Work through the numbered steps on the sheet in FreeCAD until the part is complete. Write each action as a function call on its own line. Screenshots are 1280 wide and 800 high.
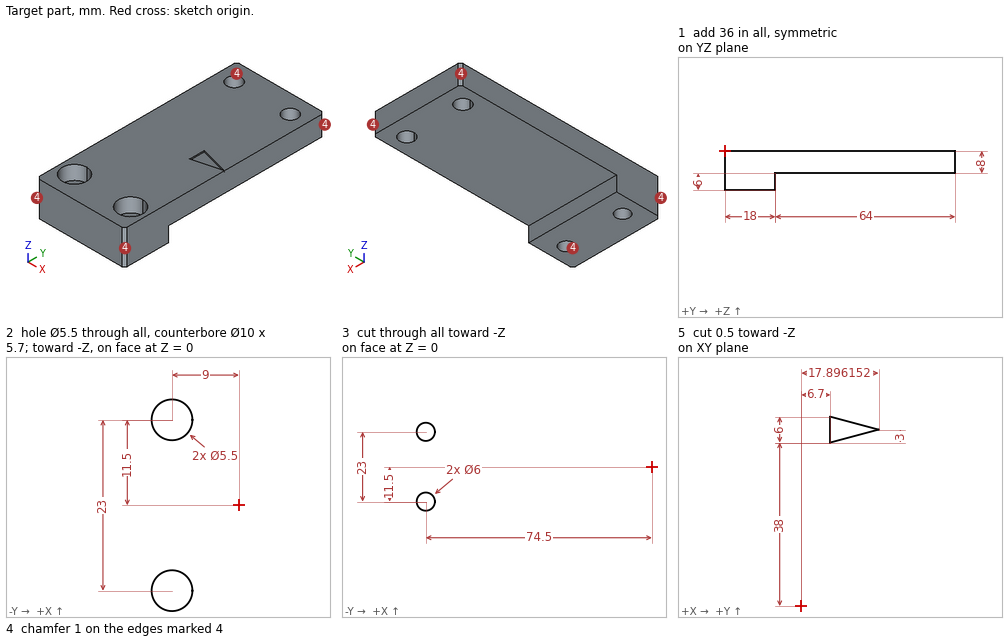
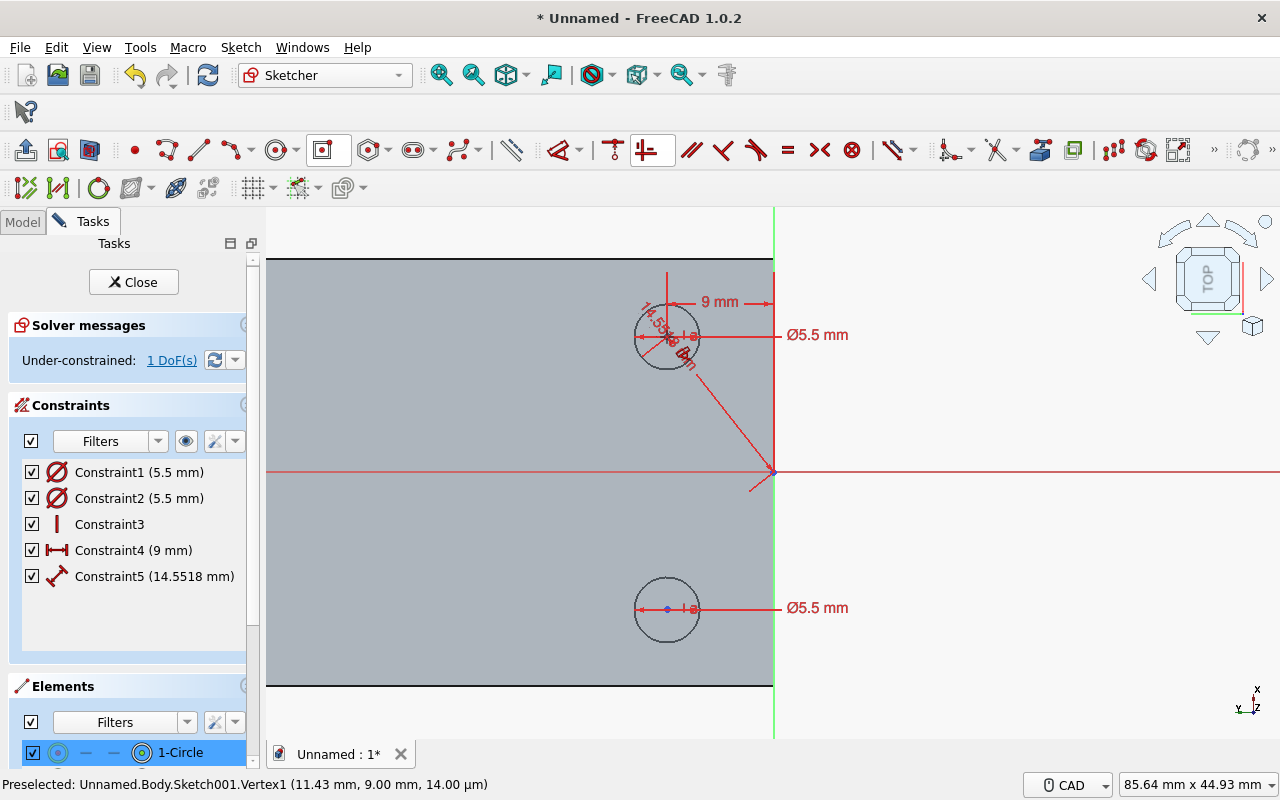
click(667, 610)
click(633, 411)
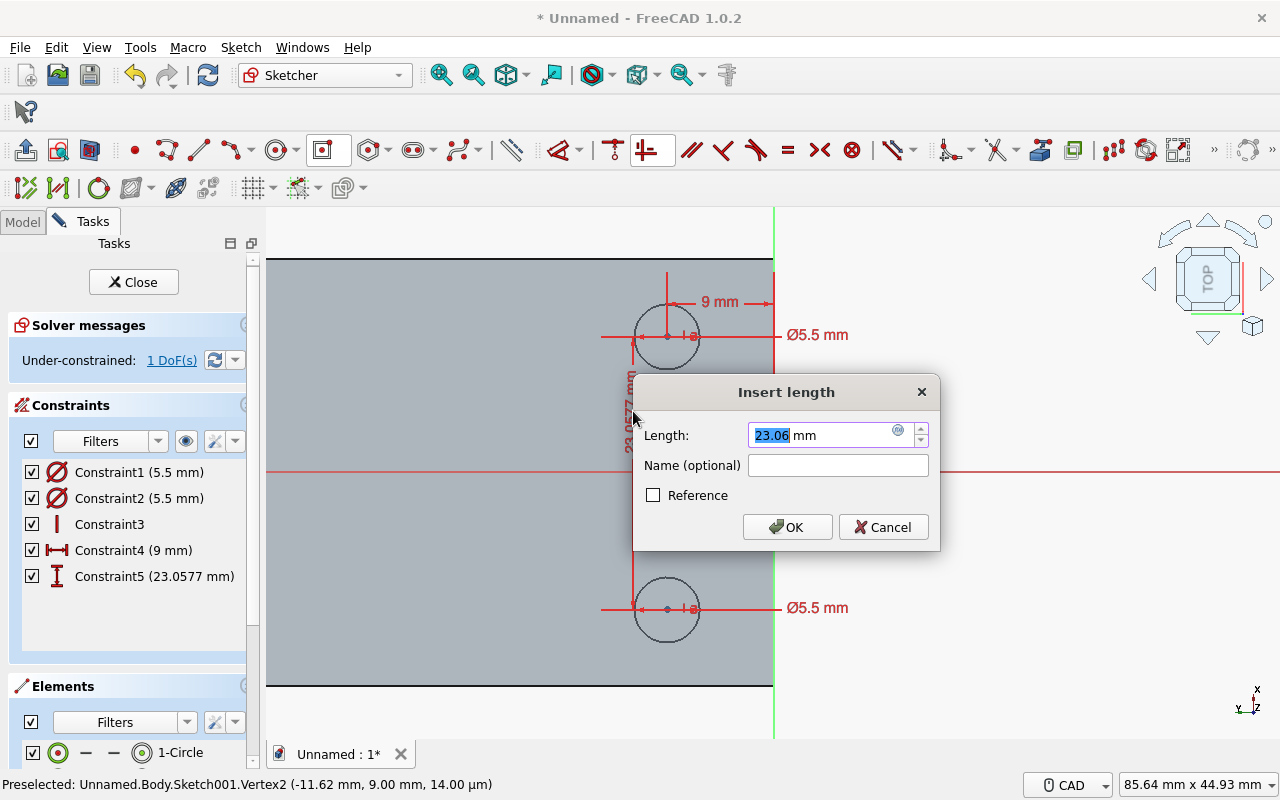
text(23)
key(Return)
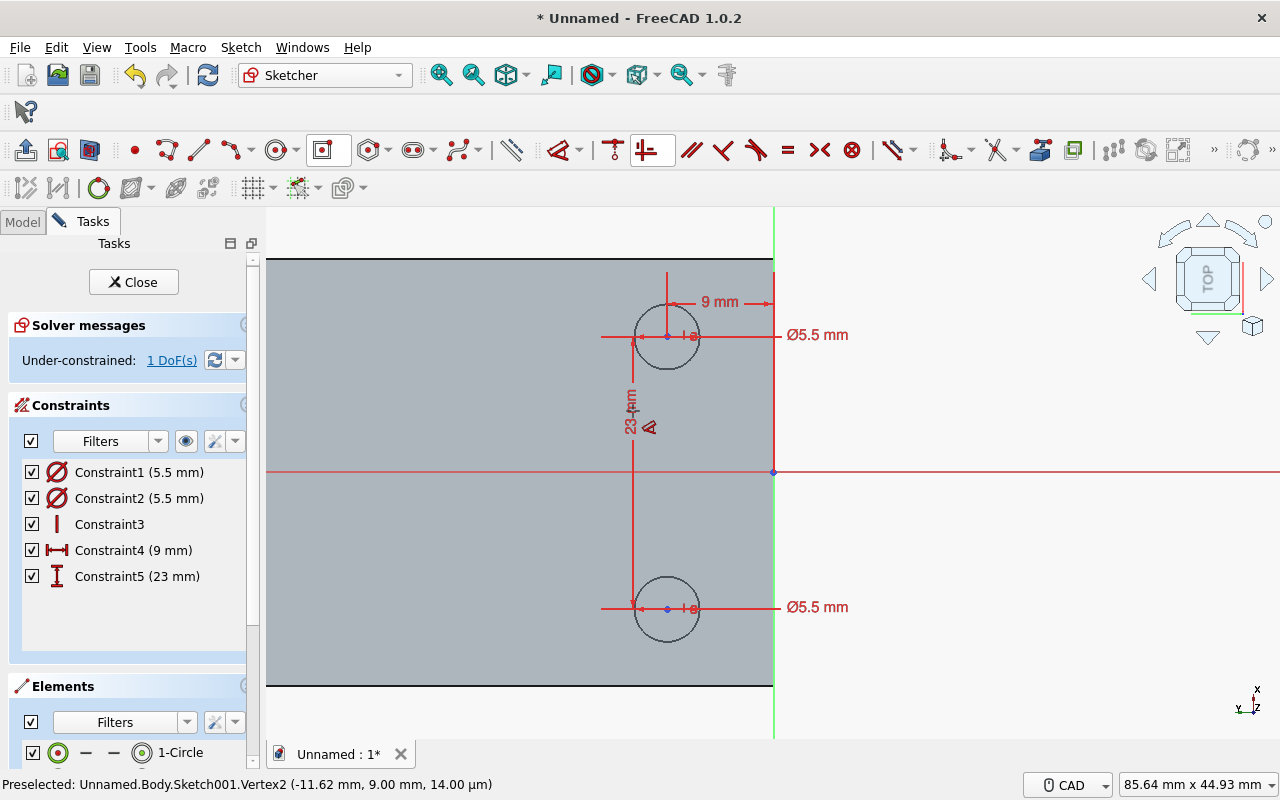
click(667, 337)
click(808, 405)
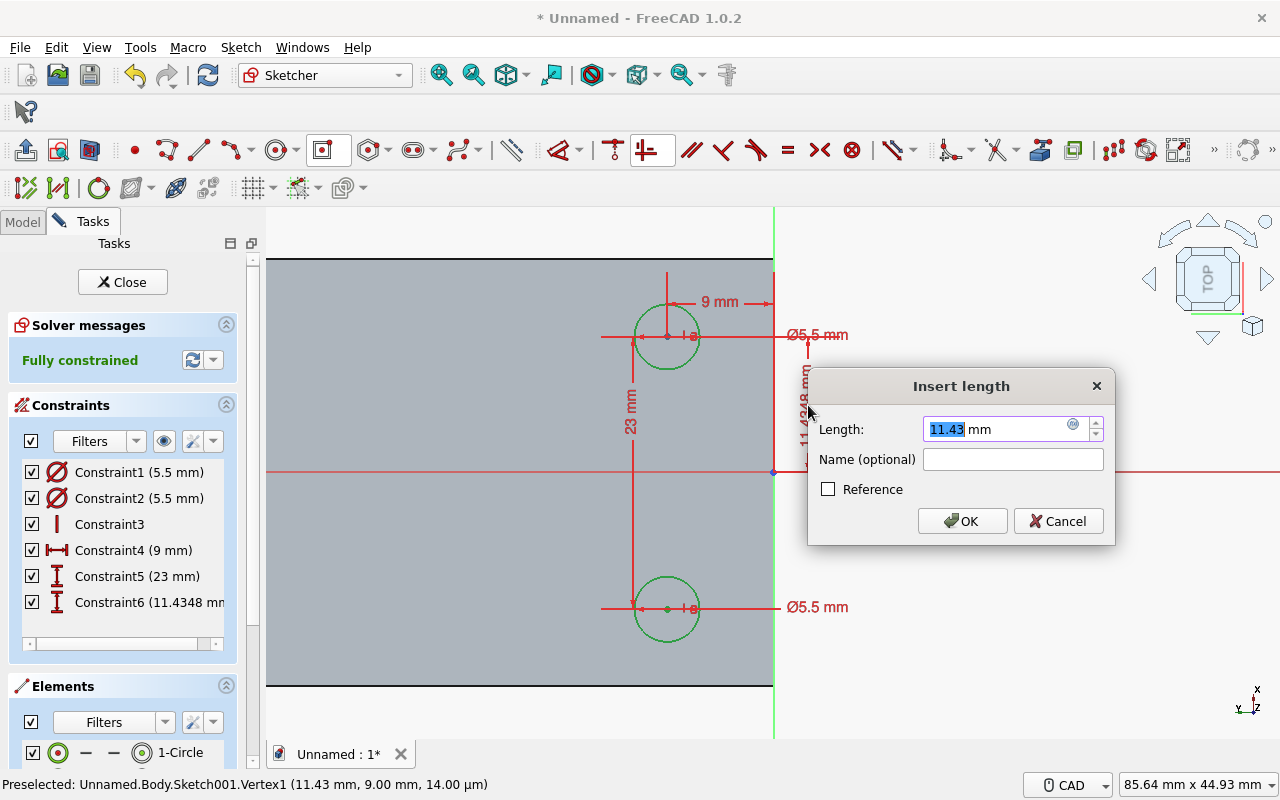
text(11.5)
key(Return)
key(Escape)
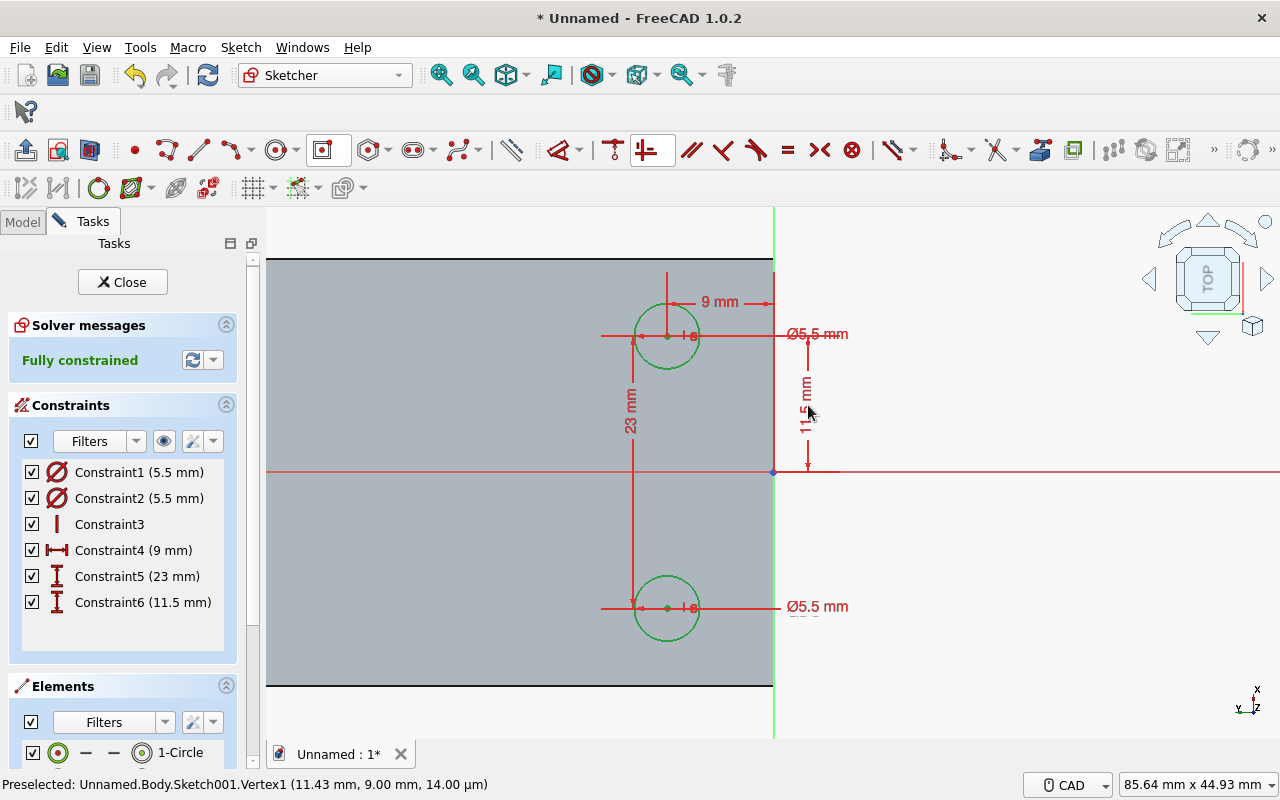
click(123, 282)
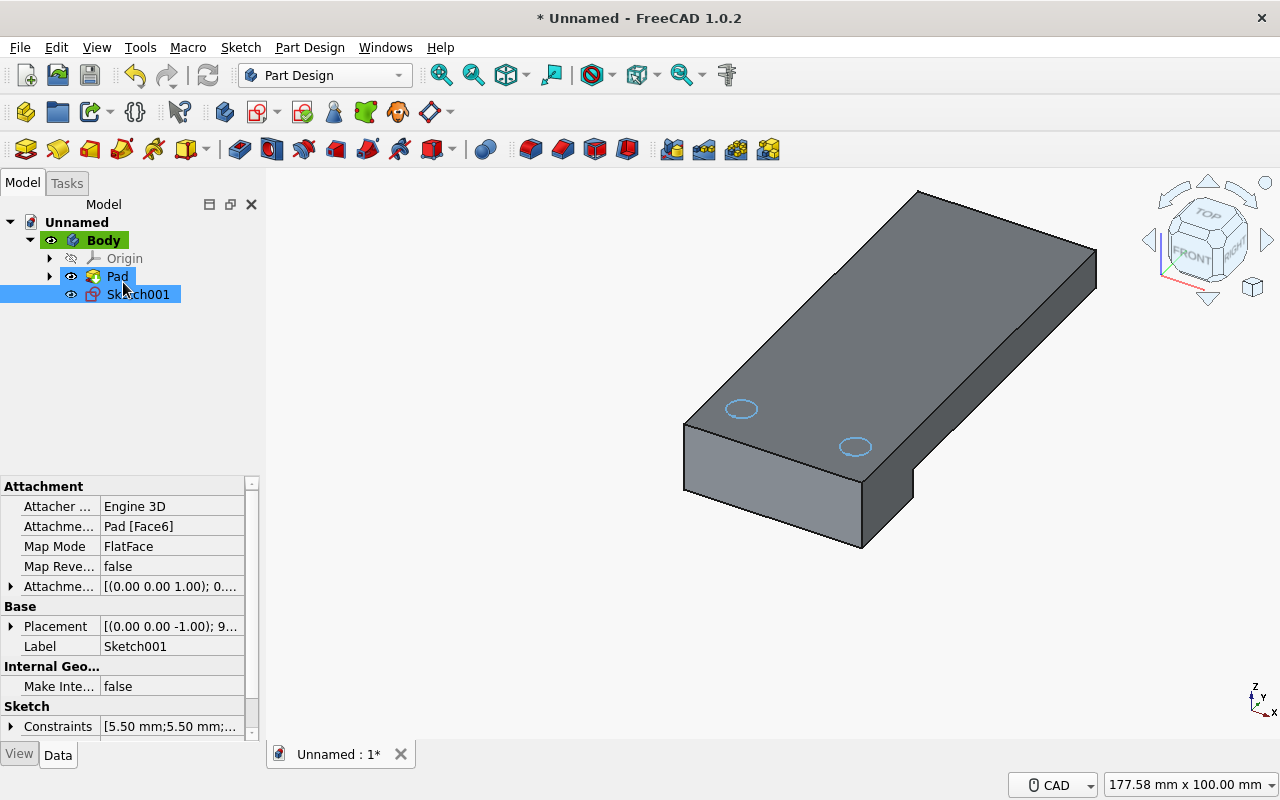
click(272, 150)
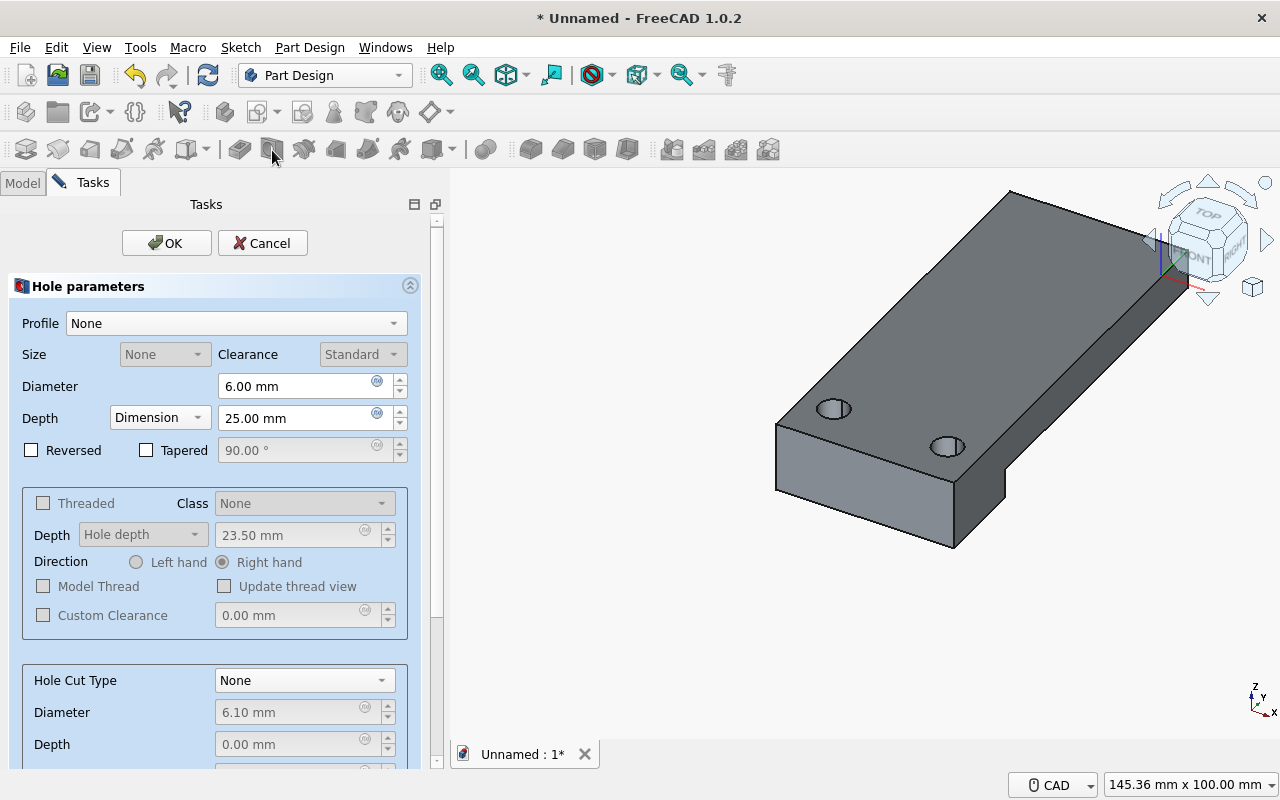
triple_click(305, 386)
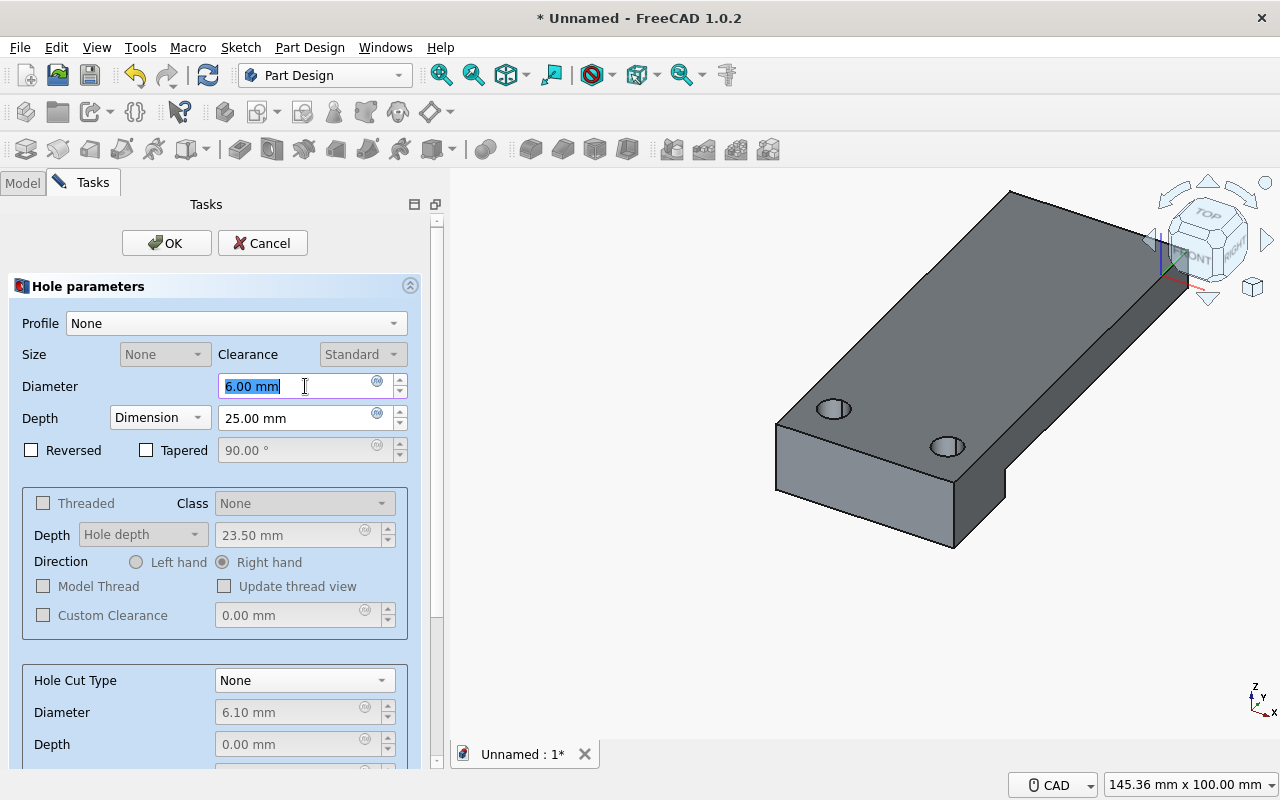
text(5.5)
key(Tab)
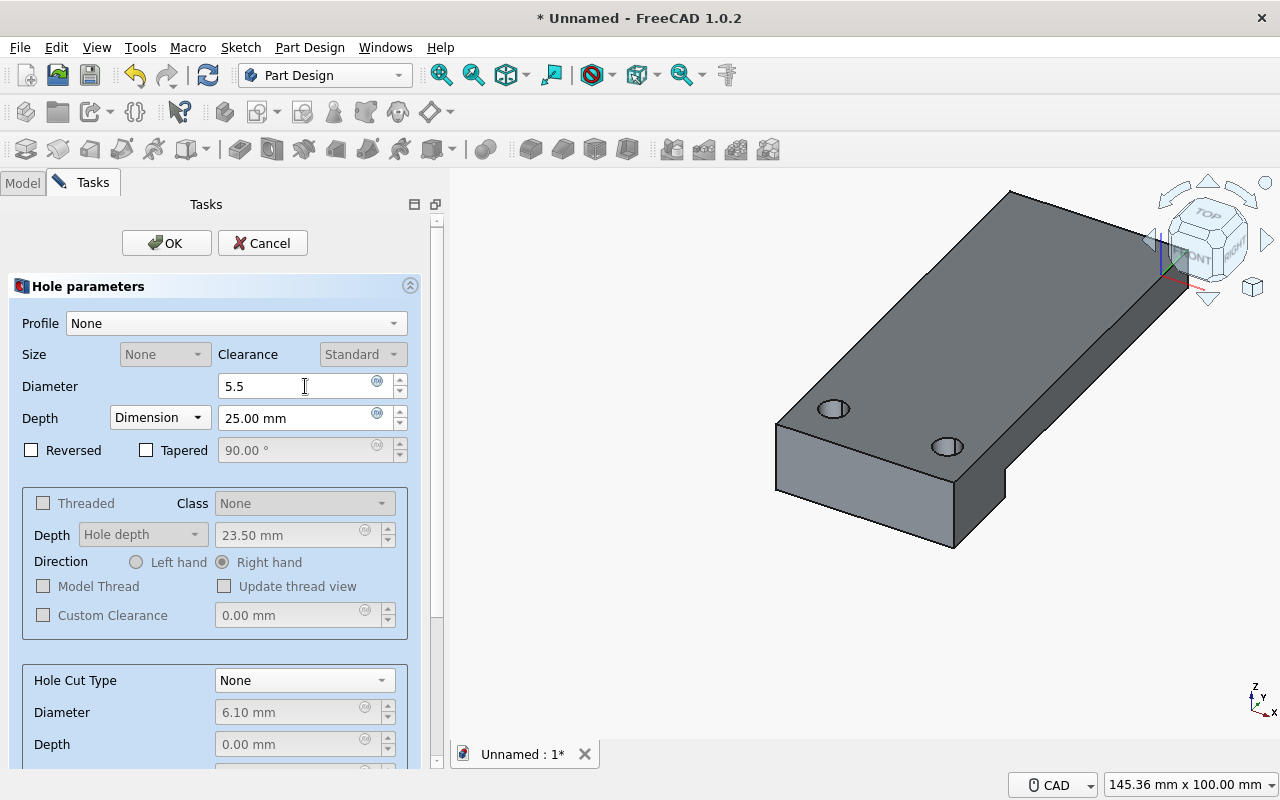
click(161, 418)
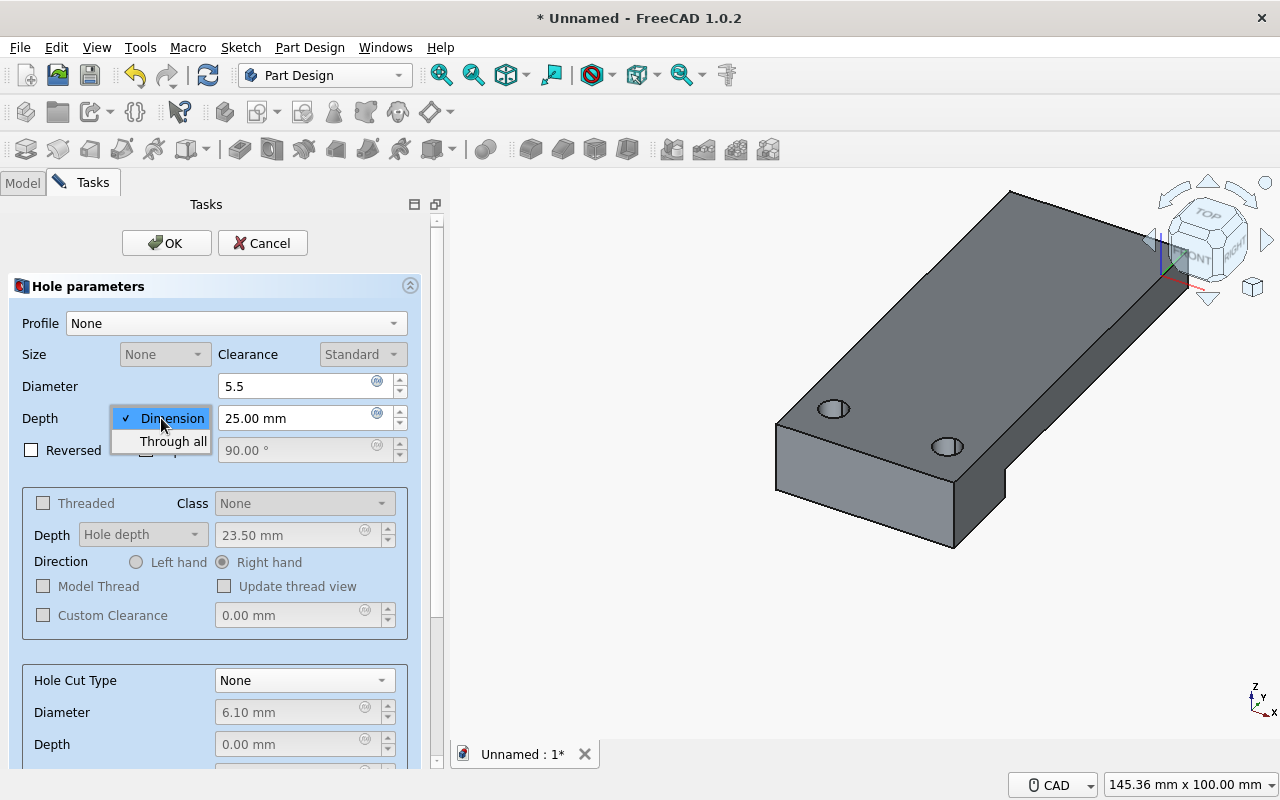
click(160, 442)